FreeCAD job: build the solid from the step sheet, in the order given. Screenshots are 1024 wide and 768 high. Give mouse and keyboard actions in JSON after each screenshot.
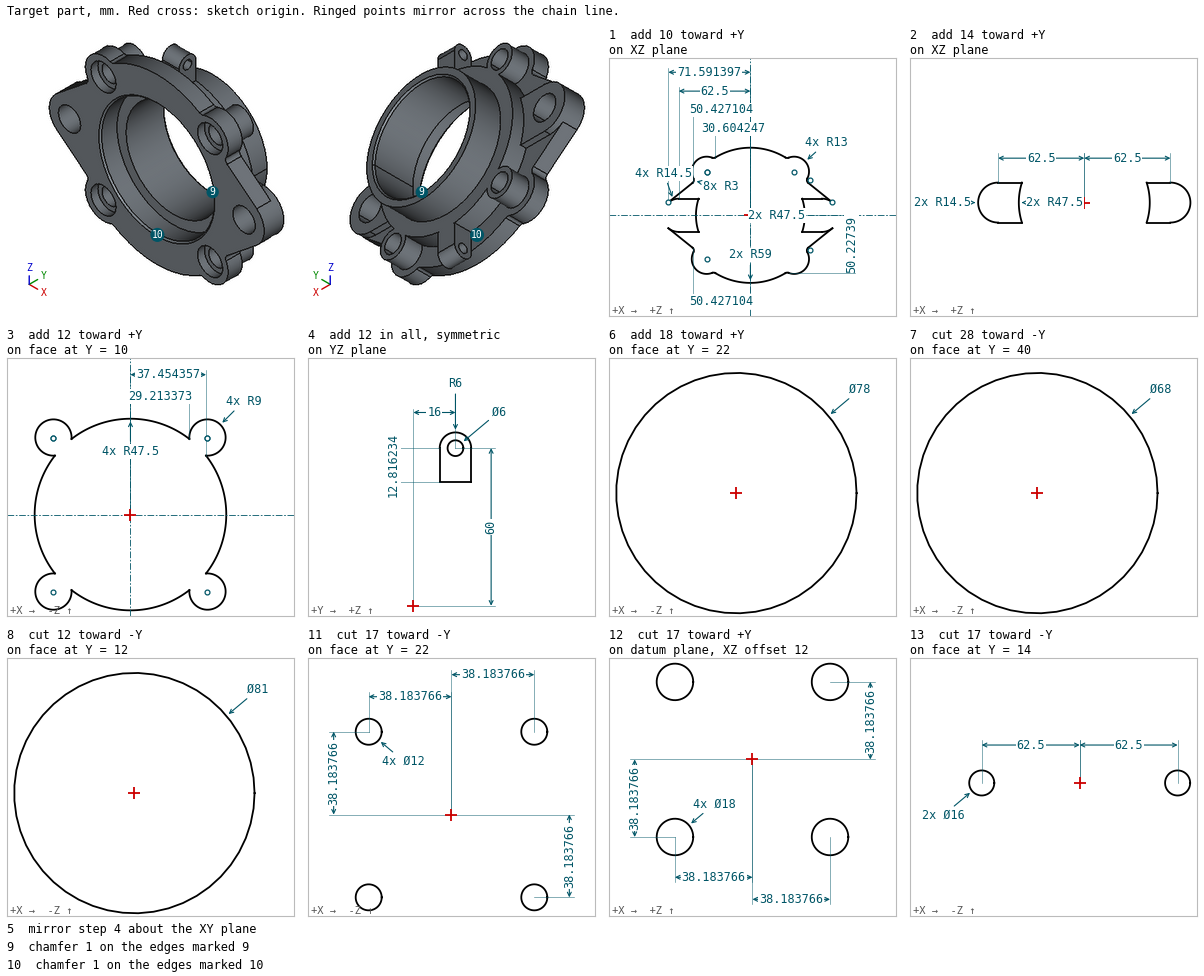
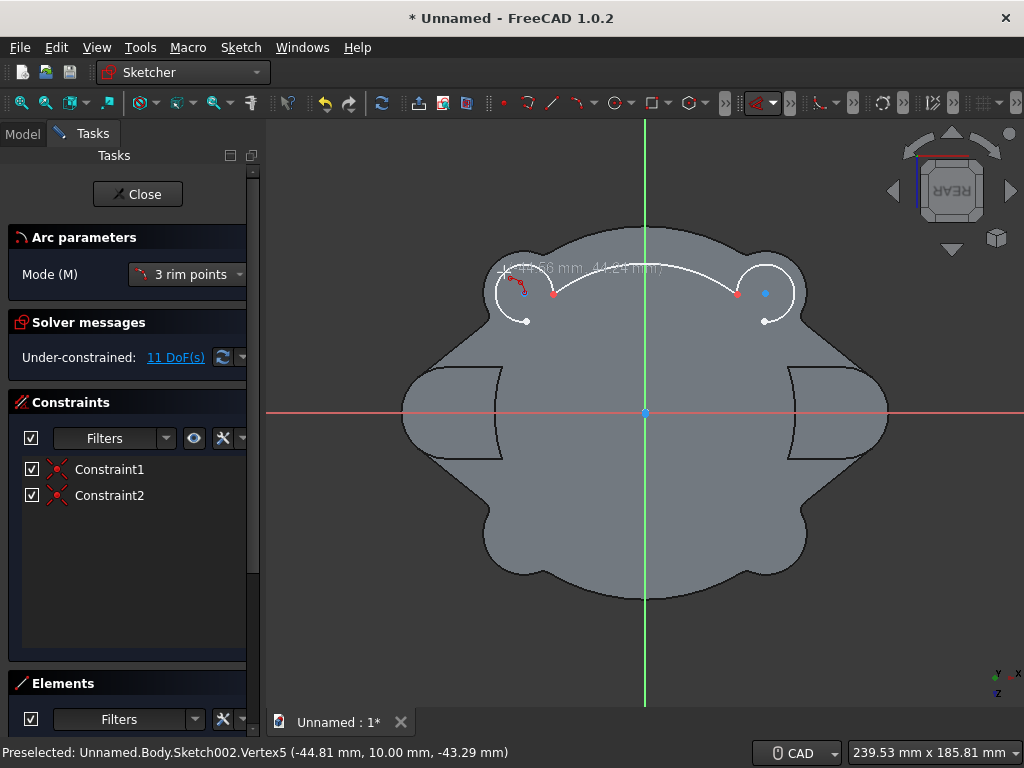
{"action": "left_click", "coordinate": [526, 322]}
{"action": "left_click", "coordinate": [526, 505]}
{"action": "left_click", "coordinate": [496, 393]}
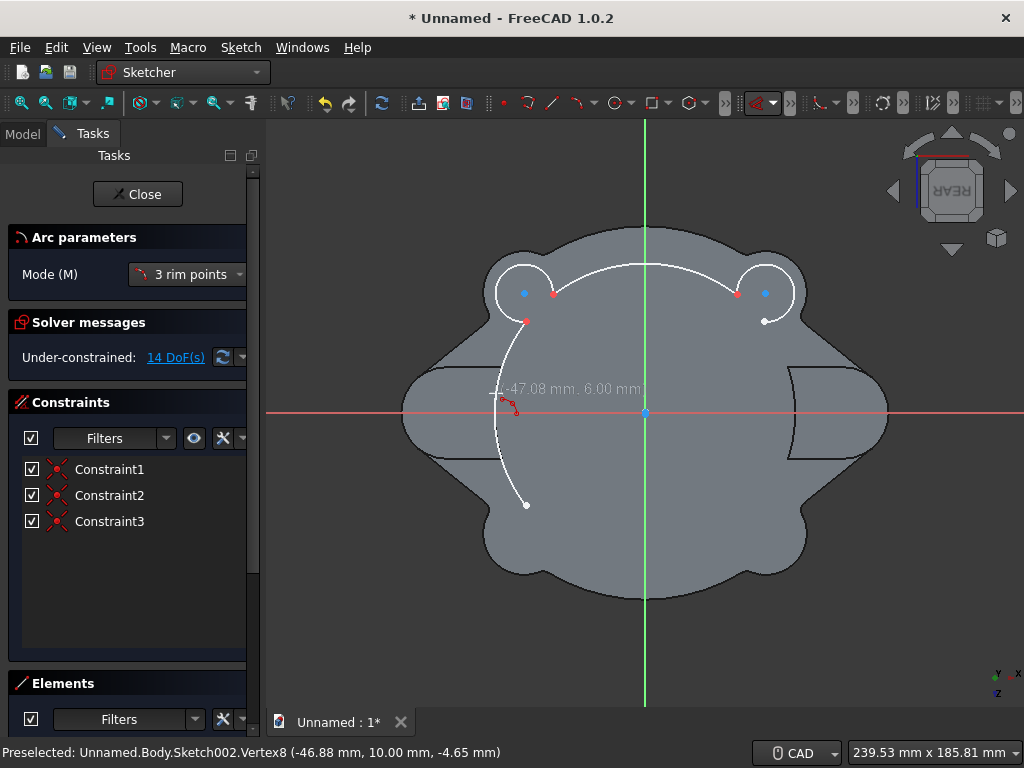
{"action": "left_click", "coordinate": [526, 506]}
{"action": "left_click", "coordinate": [553, 532]}
{"action": "left_click", "coordinate": [504, 554]}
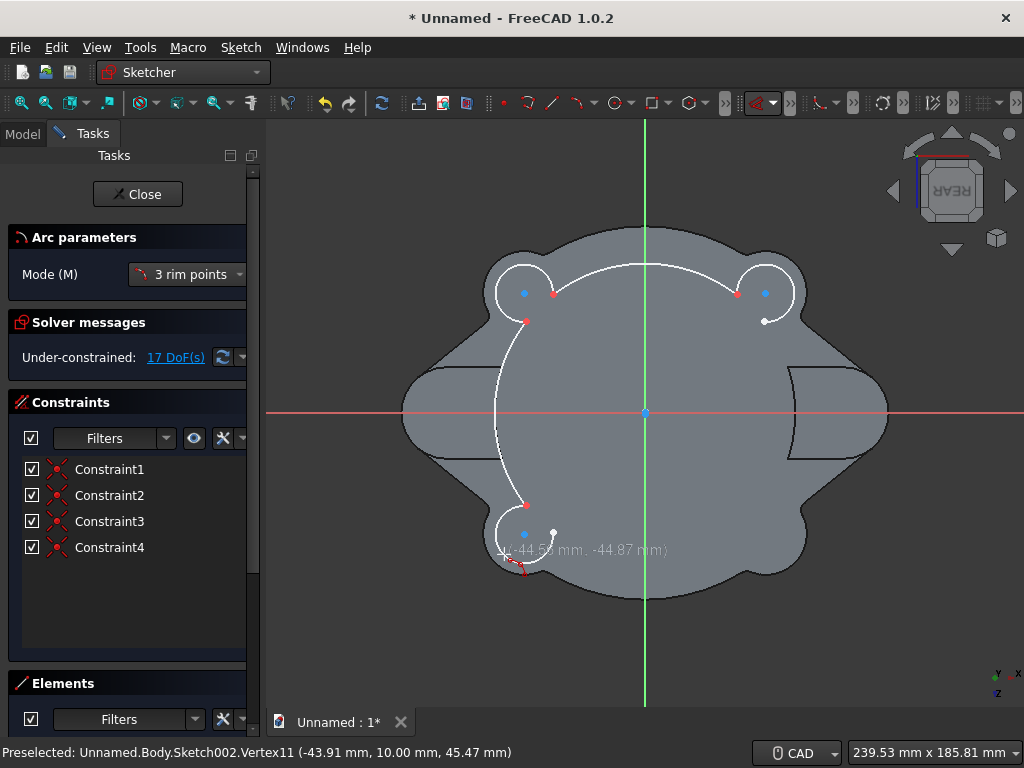
{"action": "left_click", "coordinate": [553, 533]}
{"action": "left_click", "coordinate": [737, 532]}
{"action": "left_click", "coordinate": [625, 562]}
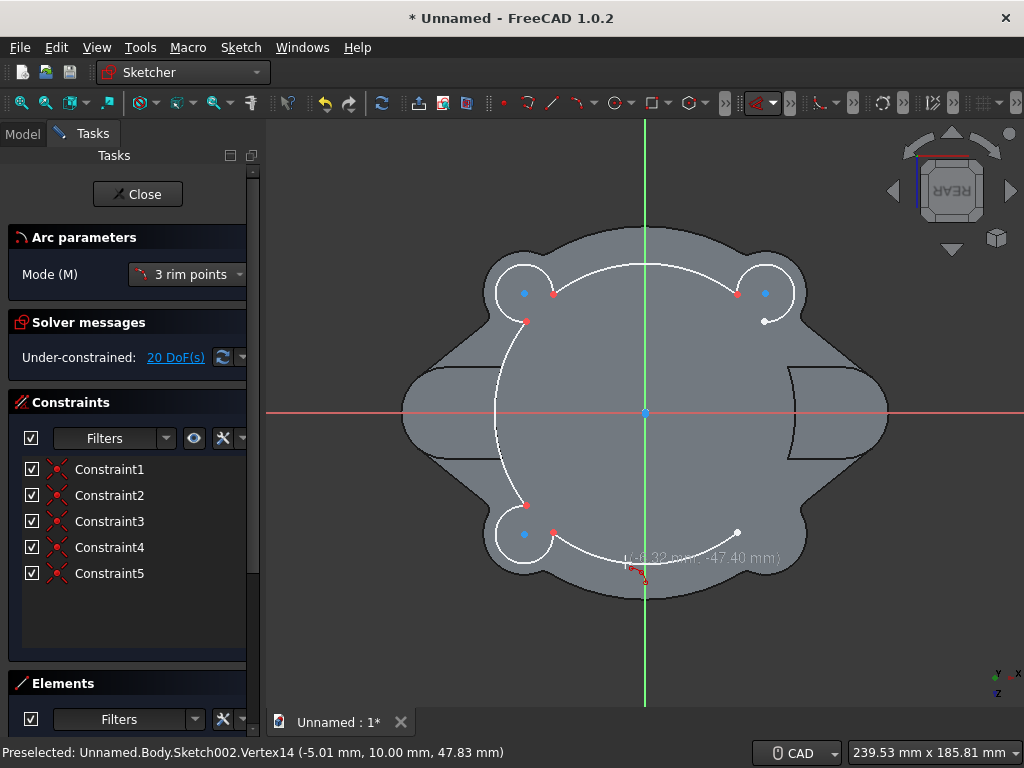
{"action": "left_click", "coordinate": [737, 533]}
{"action": "left_click", "coordinate": [764, 505]}
{"action": "left_click", "coordinate": [786, 554]}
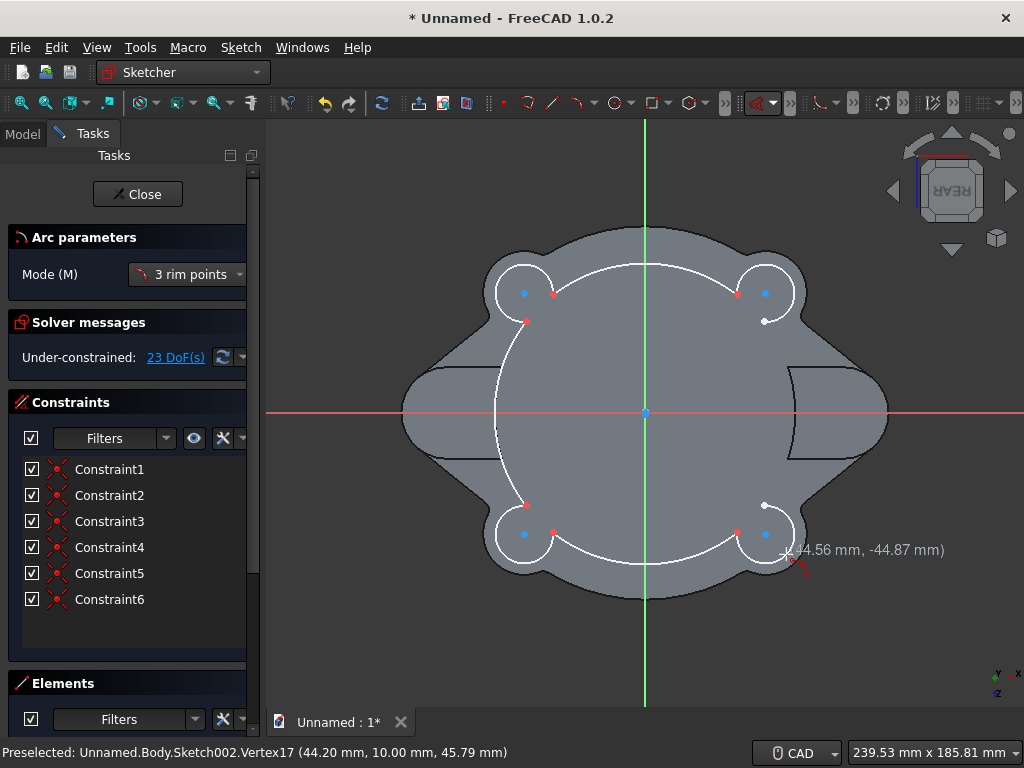
{"action": "left_click", "coordinate": [764, 506]}
{"action": "left_click", "coordinate": [764, 322]}
{"action": "left_click", "coordinate": [794, 433]}
{"action": "key", "text": "Escape"}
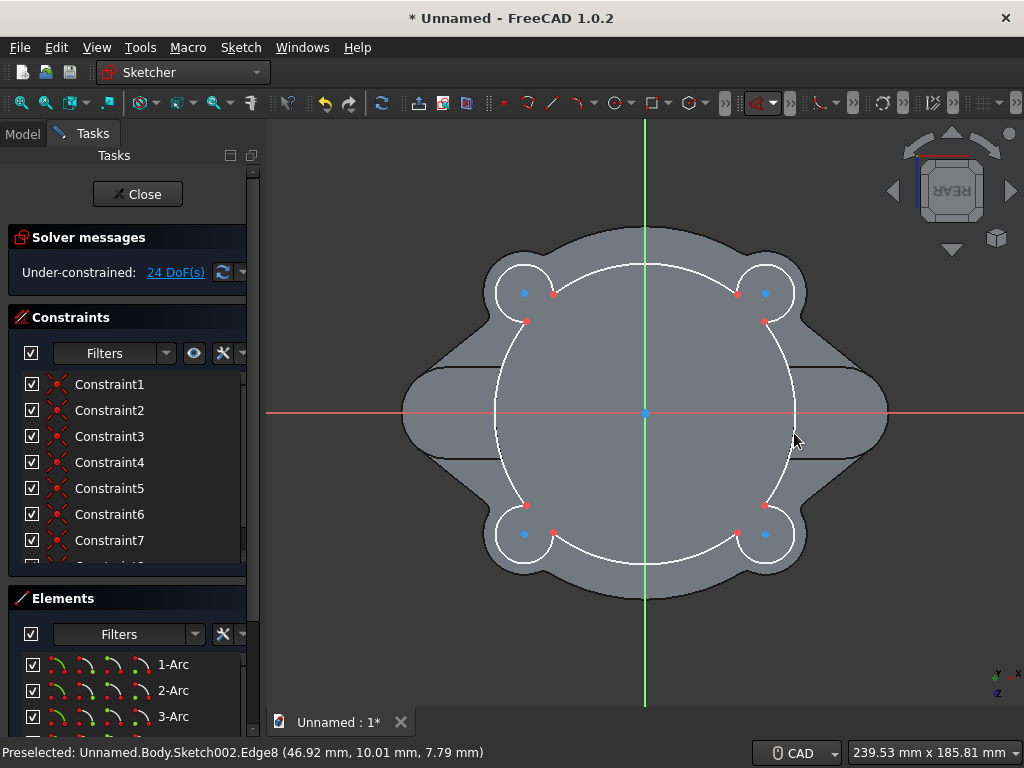
{"action": "left_click", "coordinate": [684, 269]}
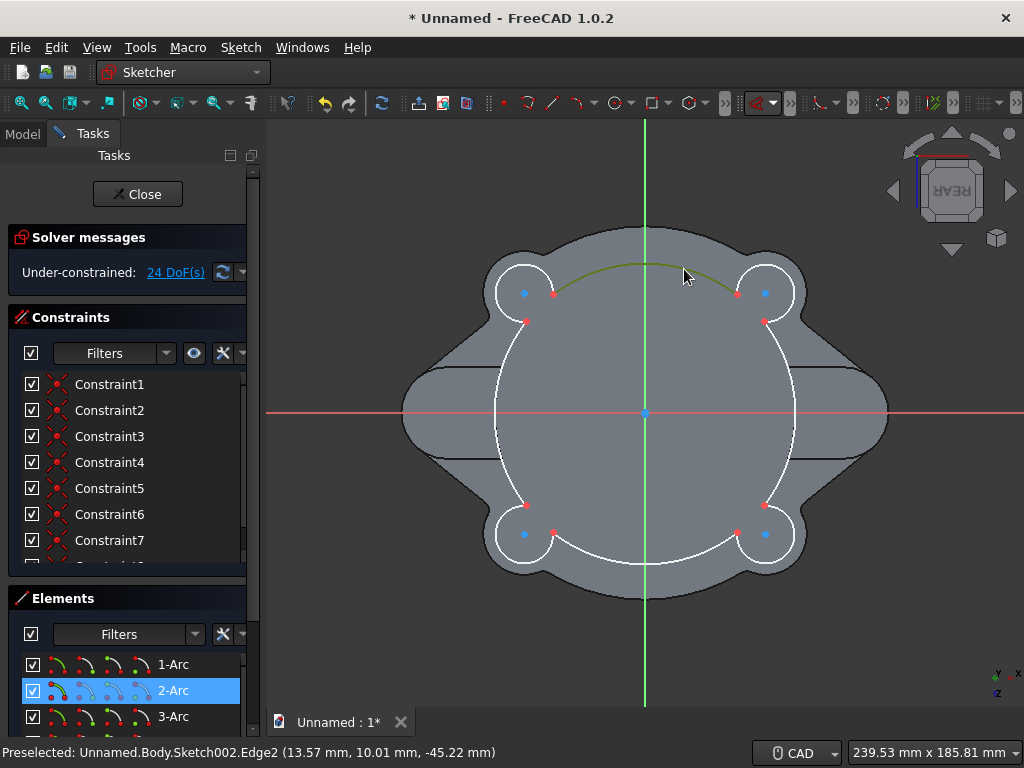
{"action": "left_click", "coordinate": [500, 375]}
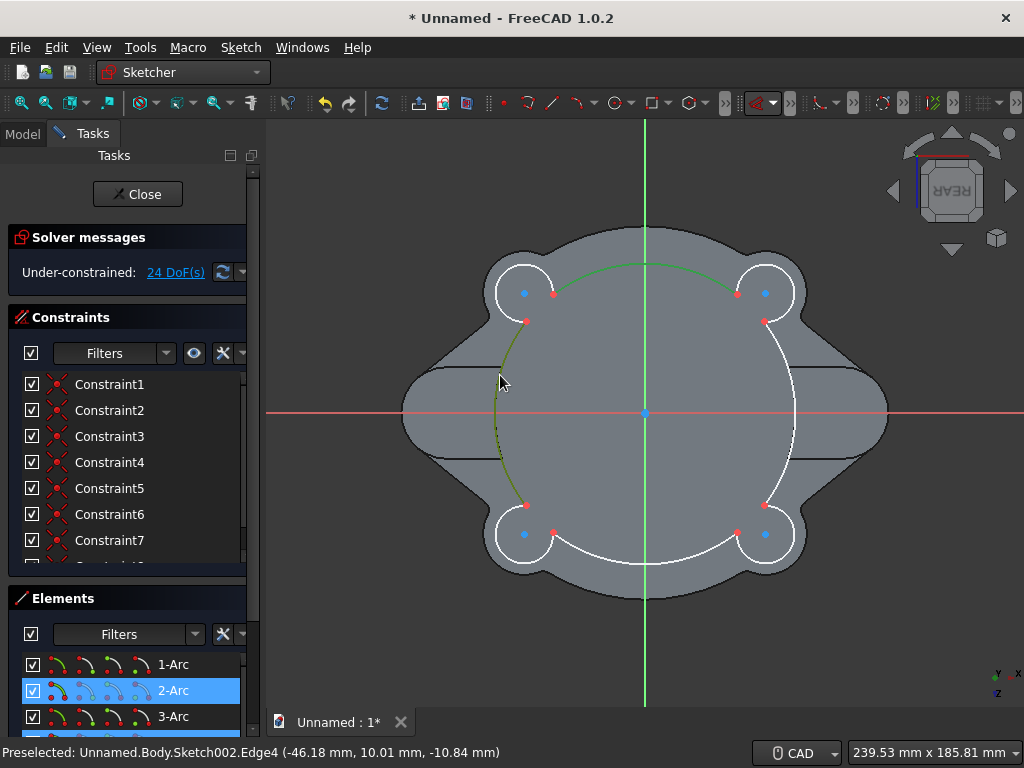
{"action": "key", "text": "c"}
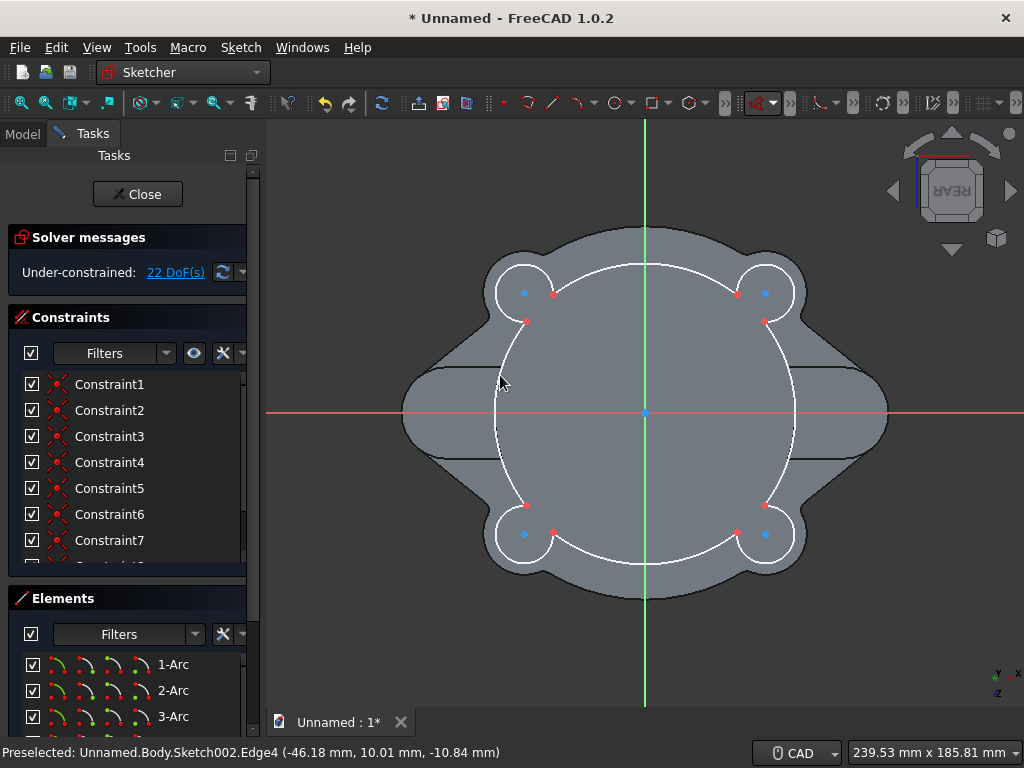
{"action": "left_click", "coordinate": [684, 269]}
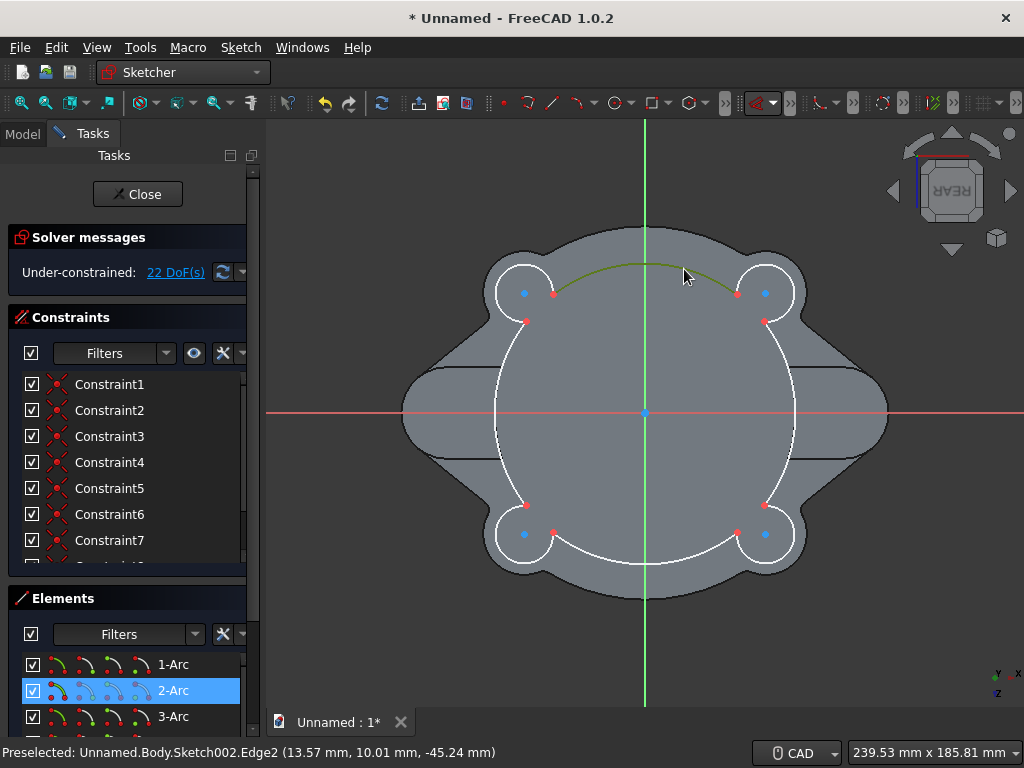
{"action": "left_click", "coordinate": [606, 559]}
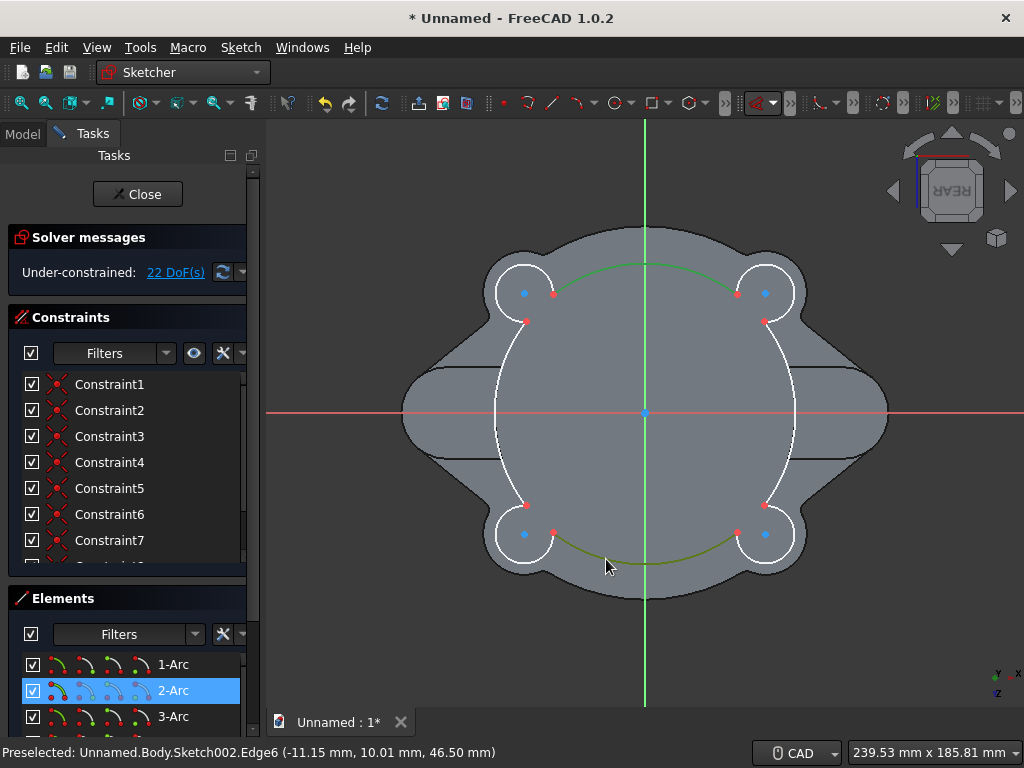
{"action": "key", "text": "c"}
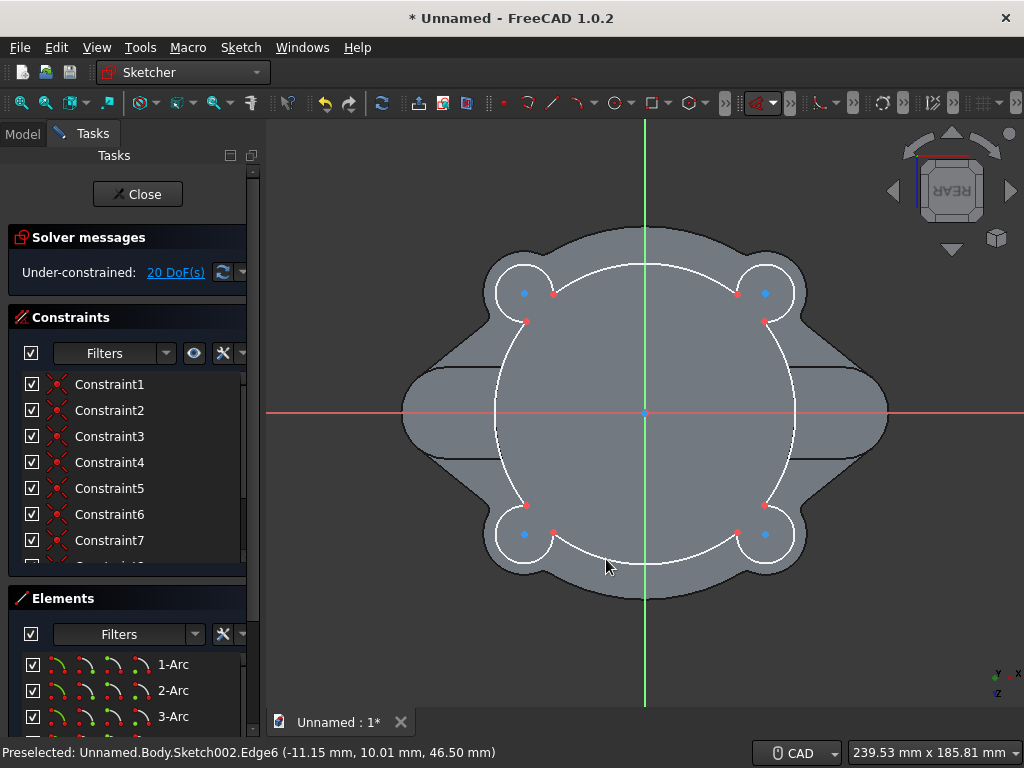
{"action": "left_click", "coordinate": [684, 269]}